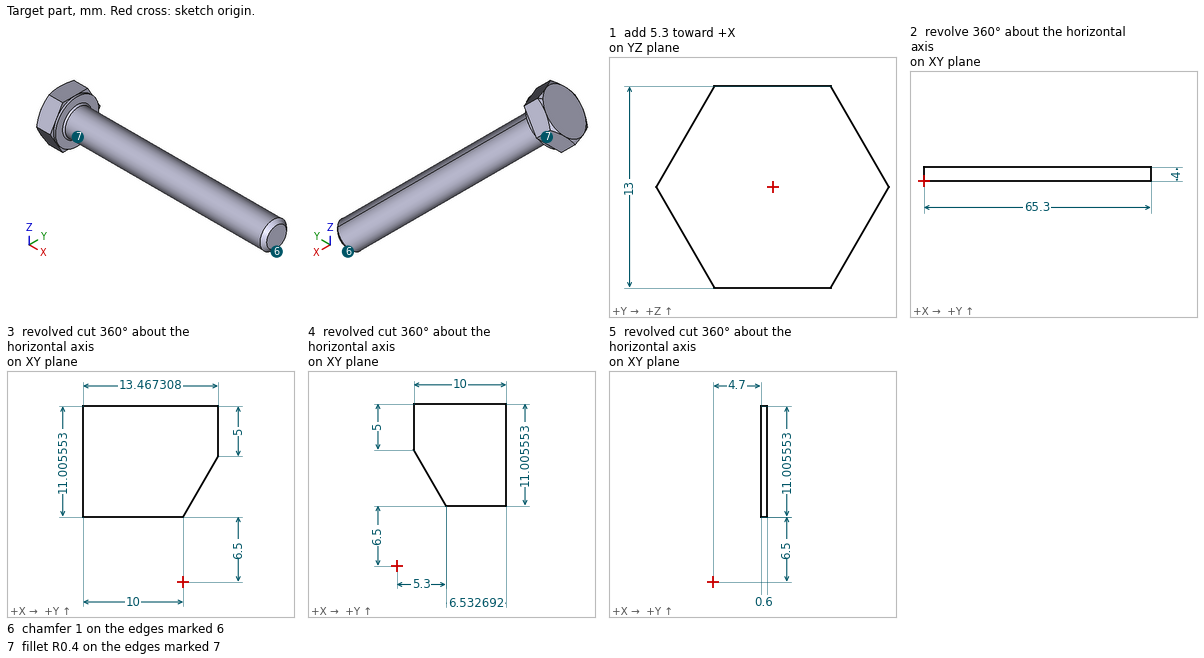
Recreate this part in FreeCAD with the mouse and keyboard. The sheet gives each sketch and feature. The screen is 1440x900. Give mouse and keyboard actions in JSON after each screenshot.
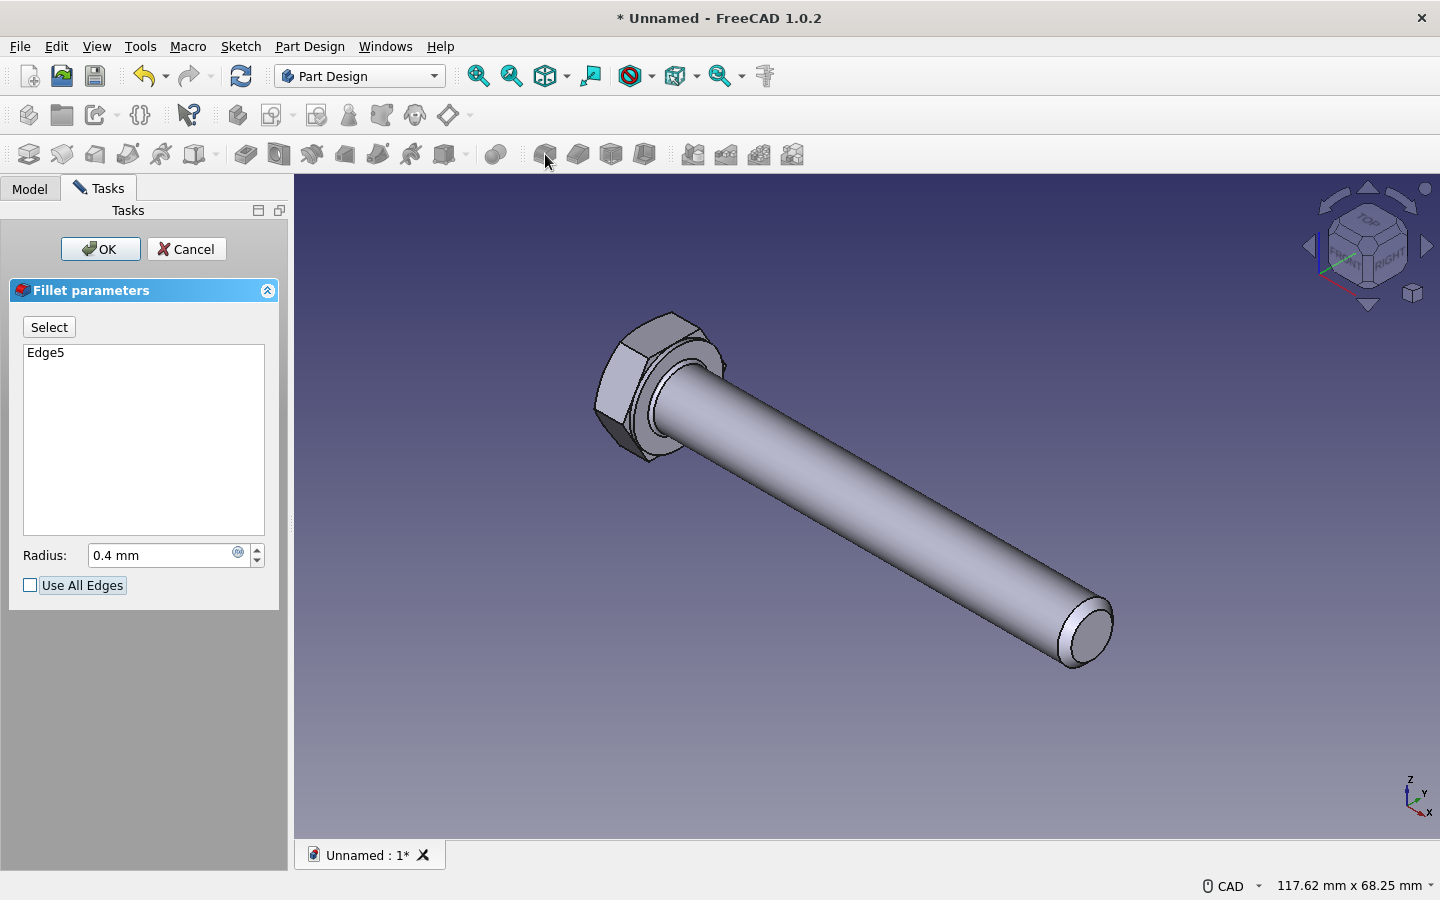
{"action": "left_click", "coordinate": [101, 249]}